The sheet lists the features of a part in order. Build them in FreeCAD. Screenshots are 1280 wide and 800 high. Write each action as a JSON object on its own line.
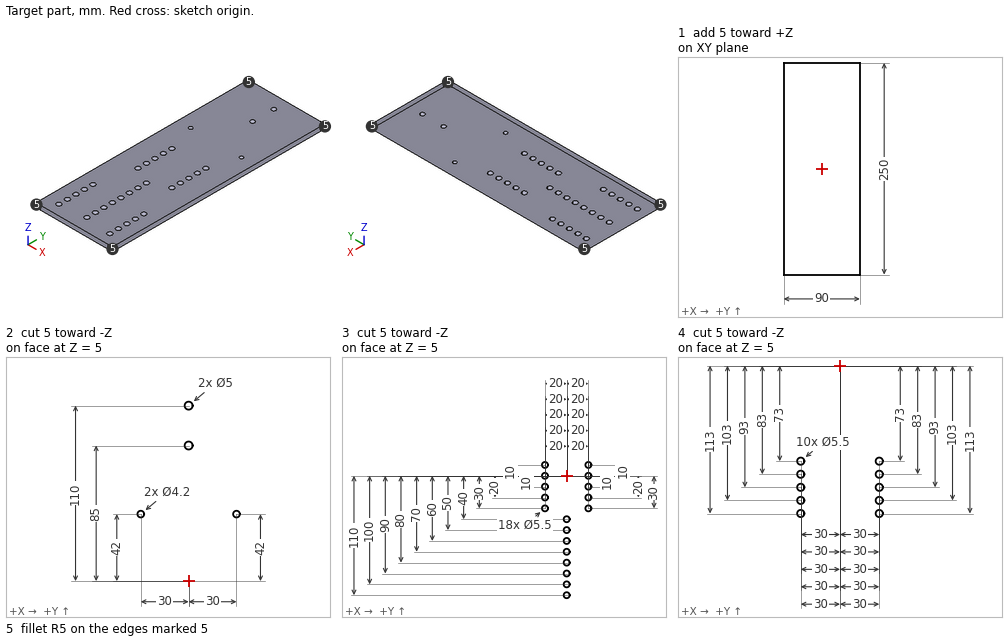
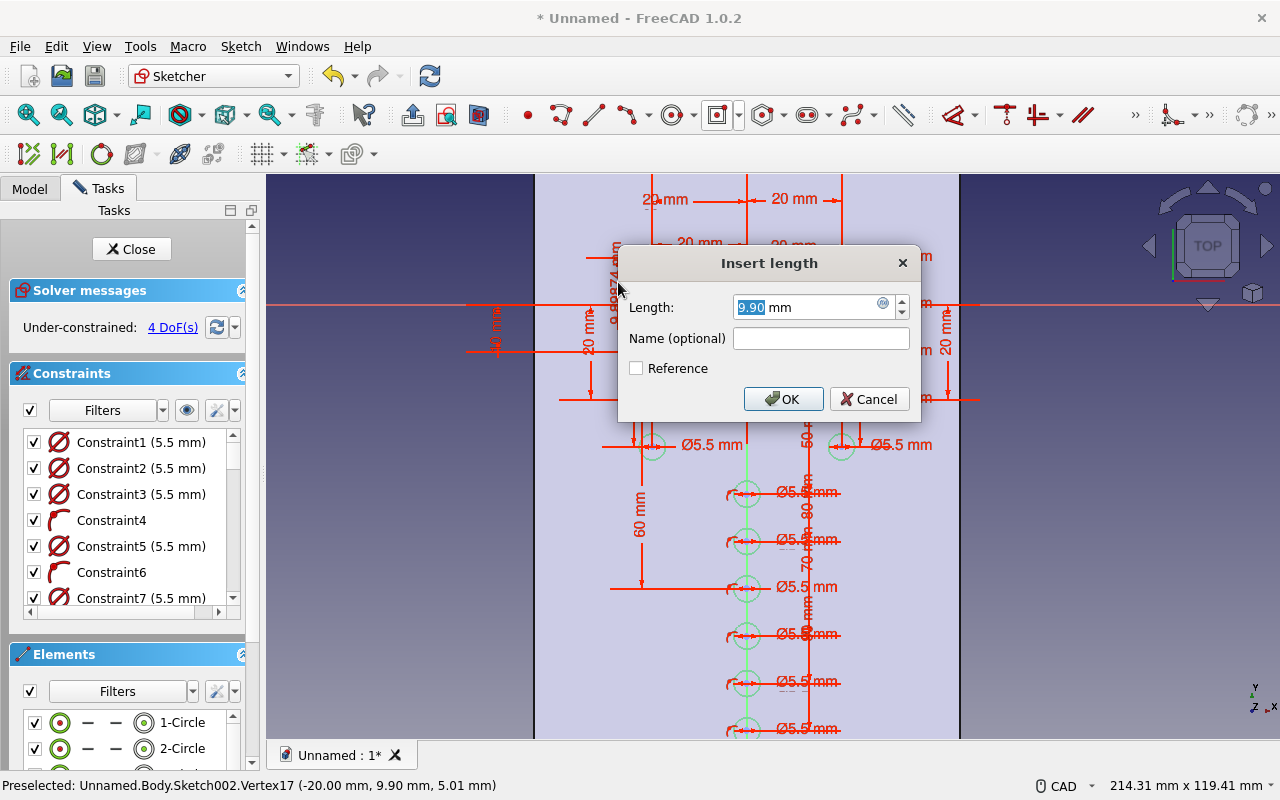
{"action": "type", "text": "10"}
{"action": "key", "text": "Return"}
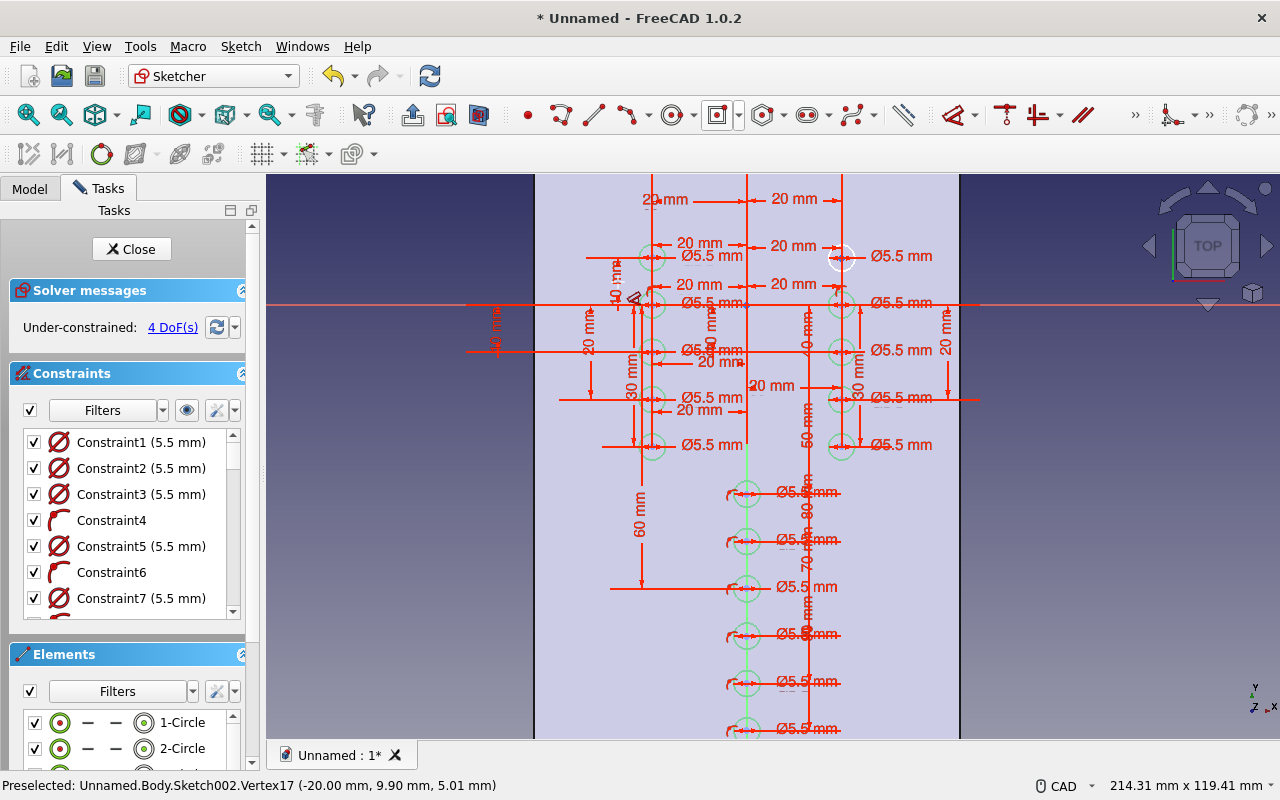
{"action": "left_click", "coordinate": [842, 258]}
{"action": "left_click", "coordinate": [794, 224]}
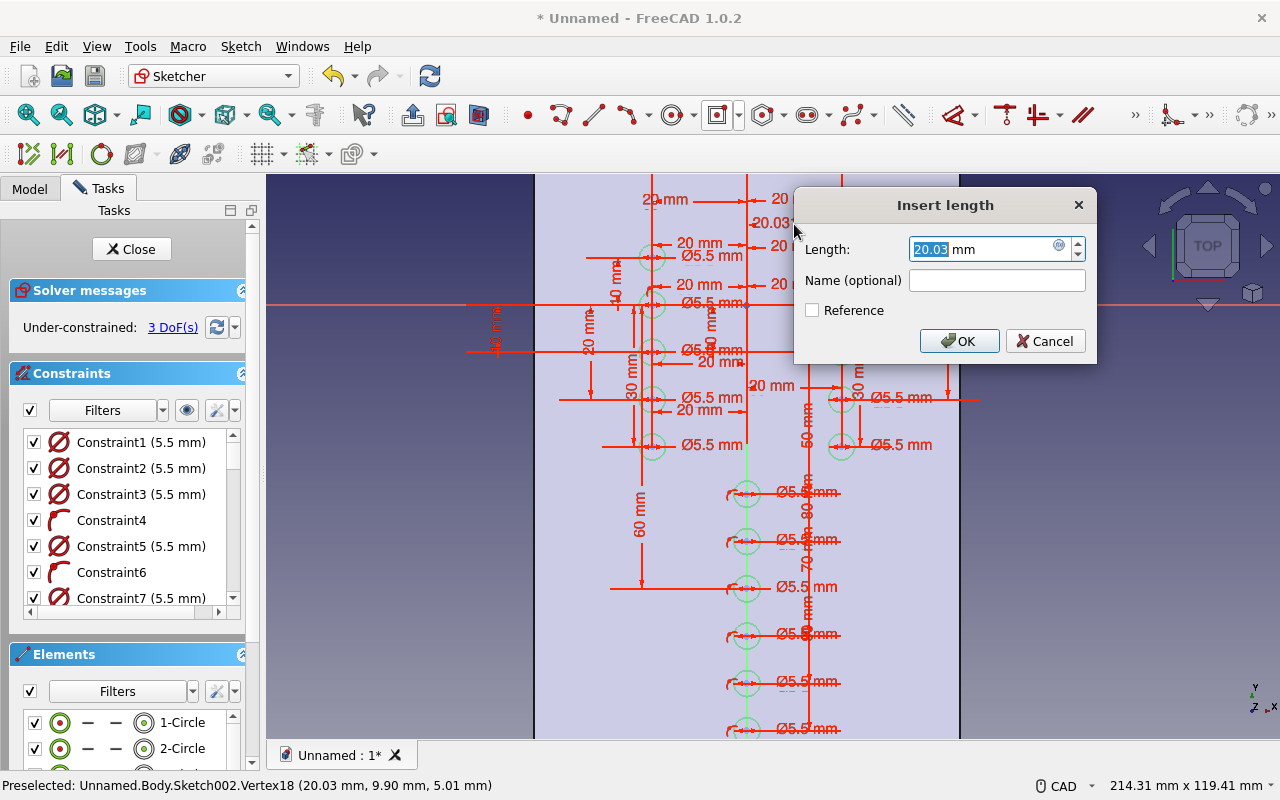
{"action": "type", "text": "20"}
{"action": "key", "text": "Return"}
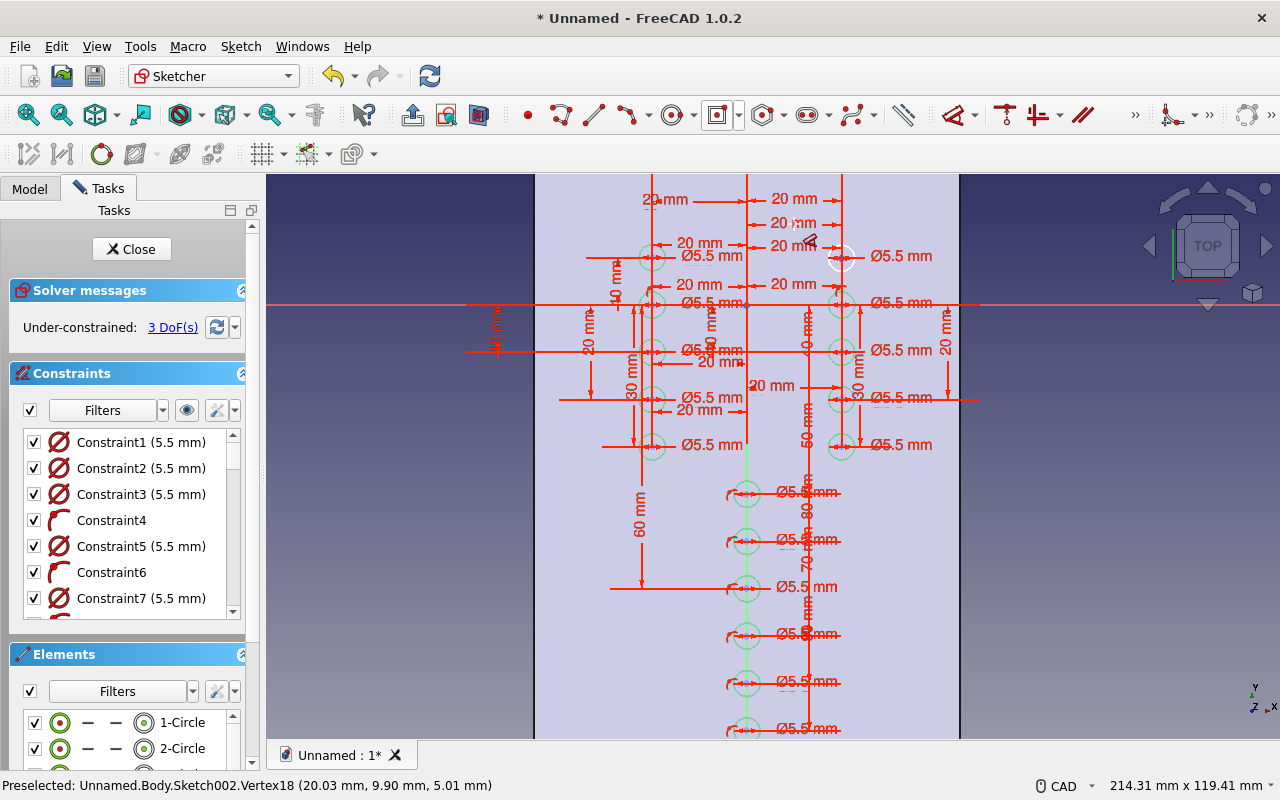
{"action": "left_click", "coordinate": [842, 258]}
{"action": "left_click", "coordinate": [876, 282]}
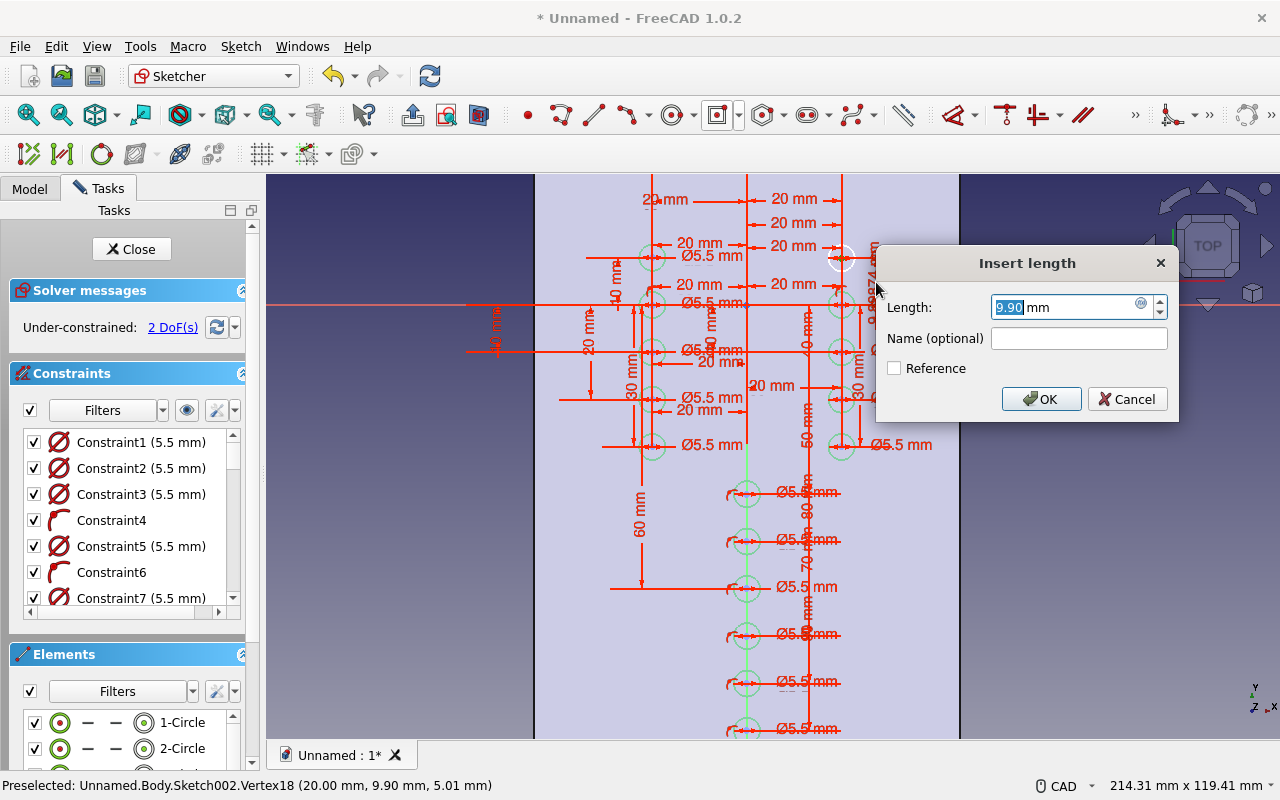
{"action": "type", "text": "10"}
{"action": "key", "text": "Return"}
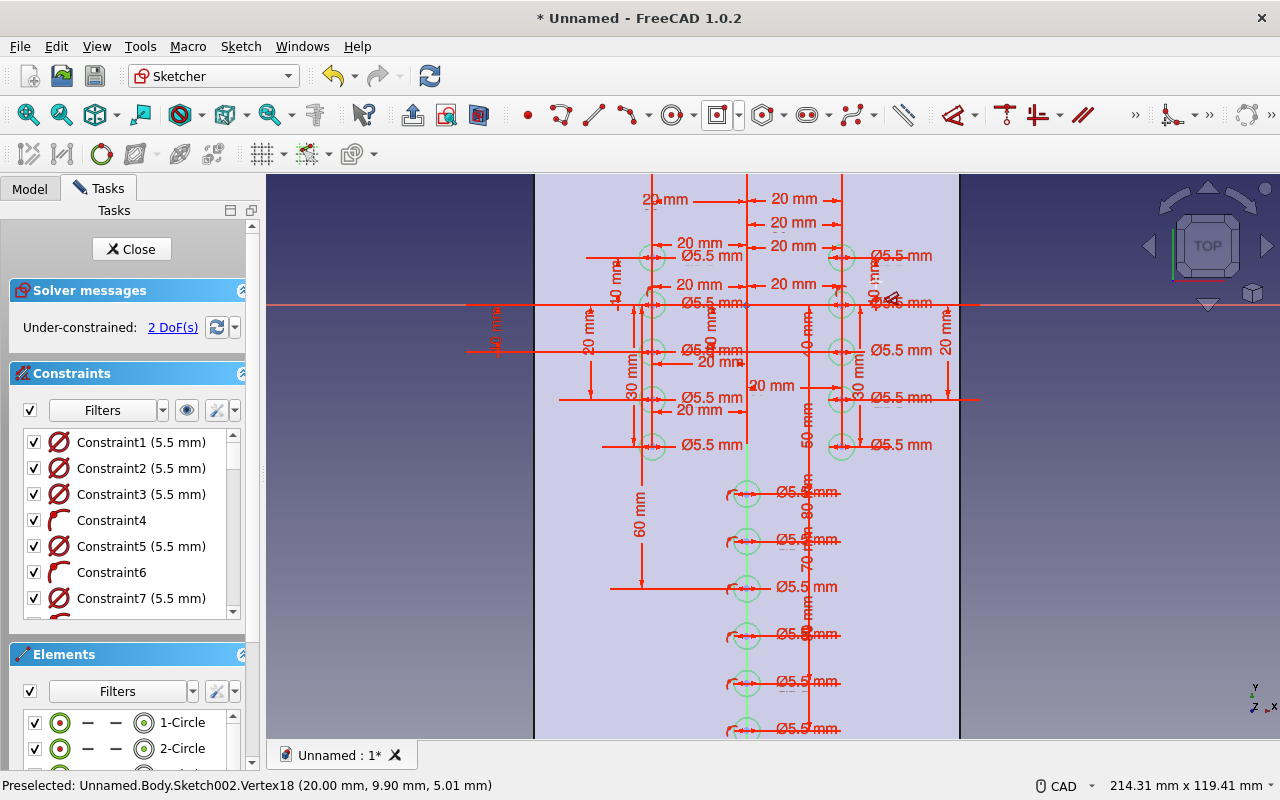
{"action": "scroll", "coordinate": [653, 353], "scroll_direction": "down", "scroll_amount": 3}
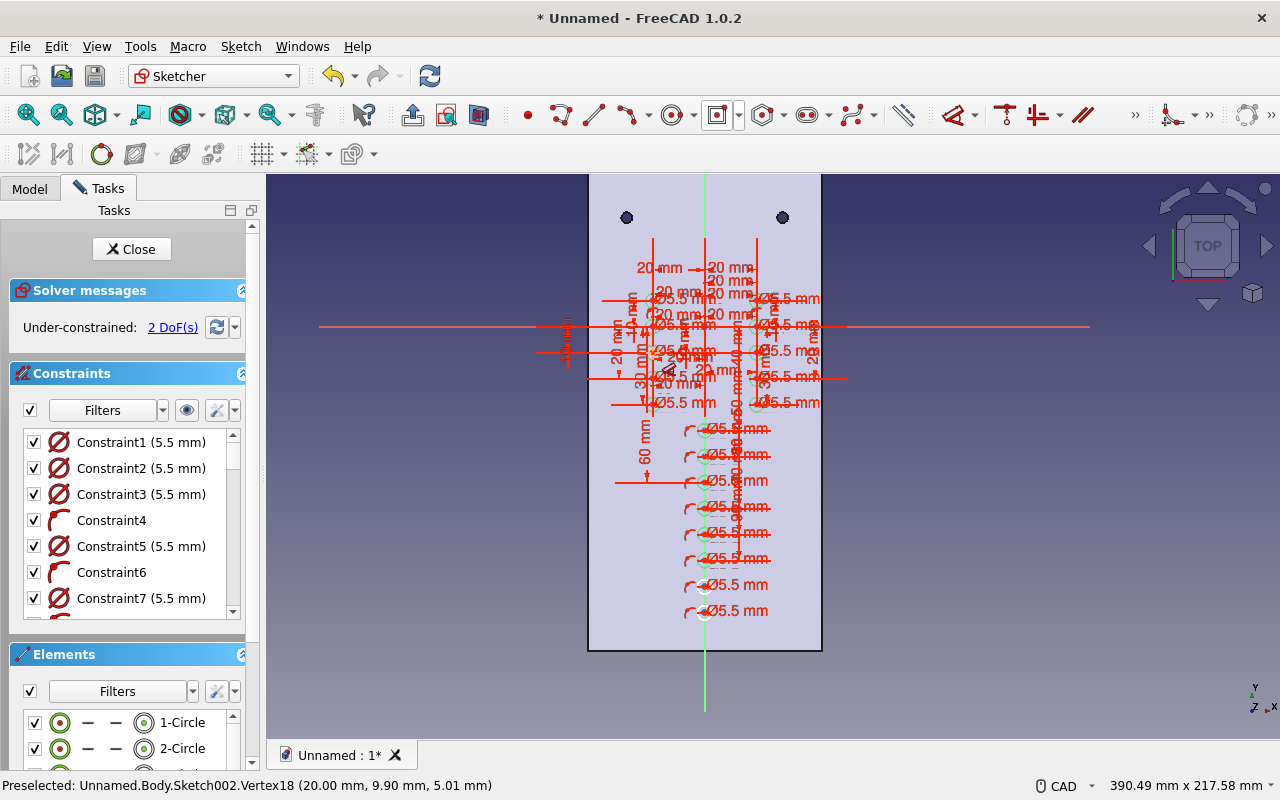
{"action": "left_click", "coordinate": [705, 587]}
{"action": "left_click", "coordinate": [739, 548]}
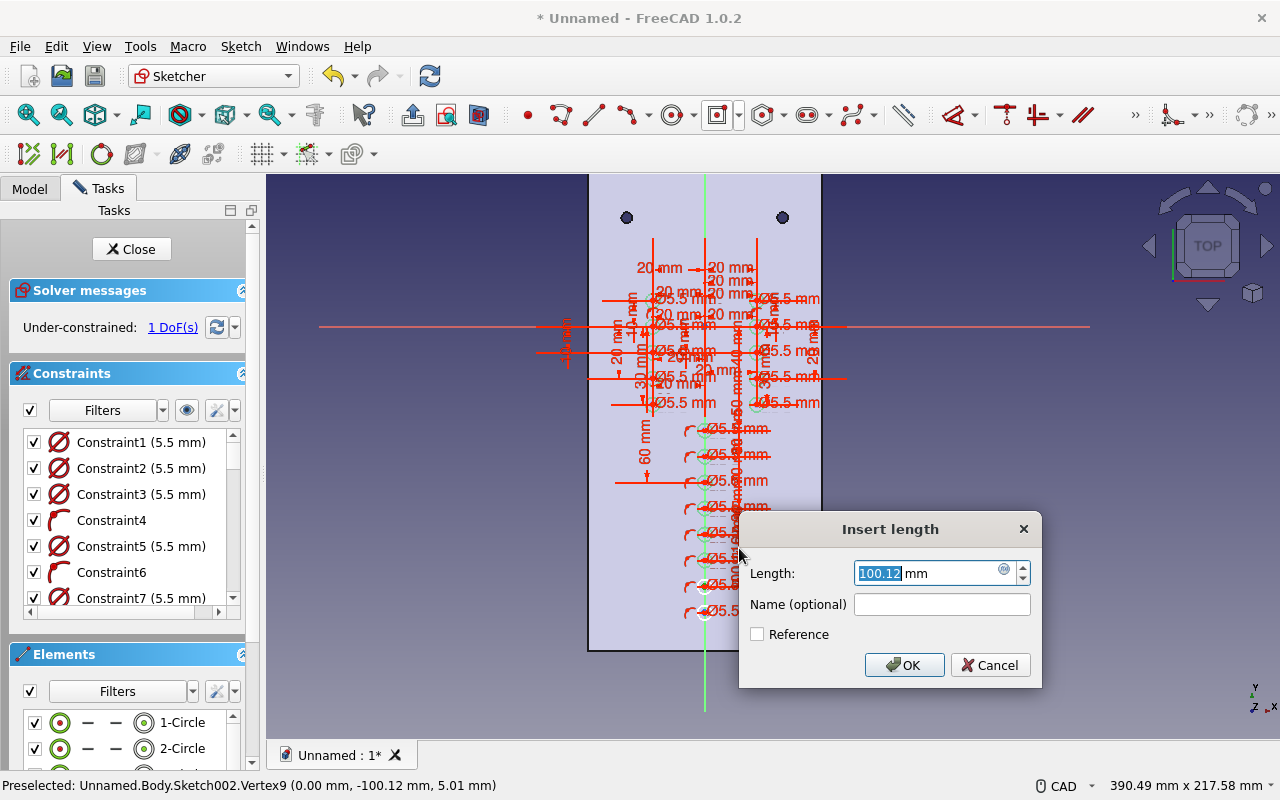
{"action": "type", "text": "100"}
{"action": "key", "text": "Return"}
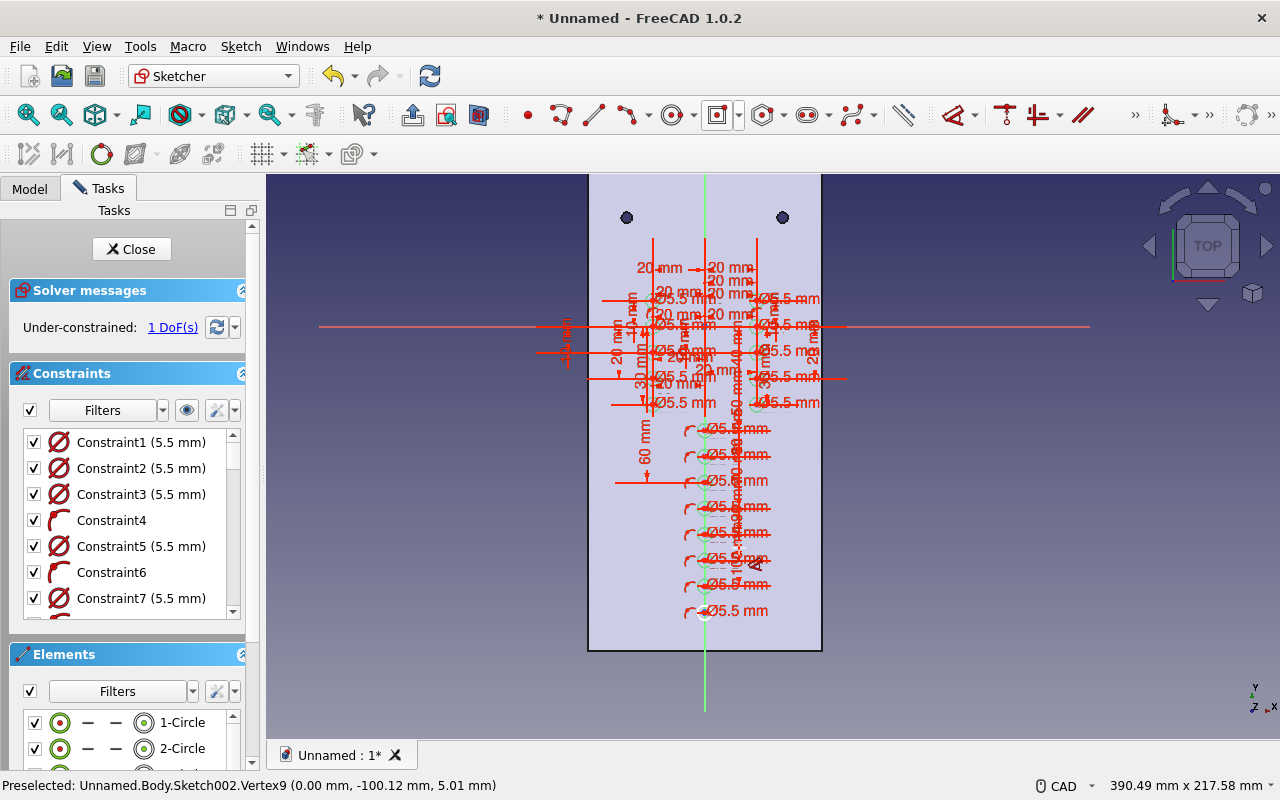
{"action": "left_click", "coordinate": [705, 613]}
{"action": "left_click", "coordinate": [739, 570]}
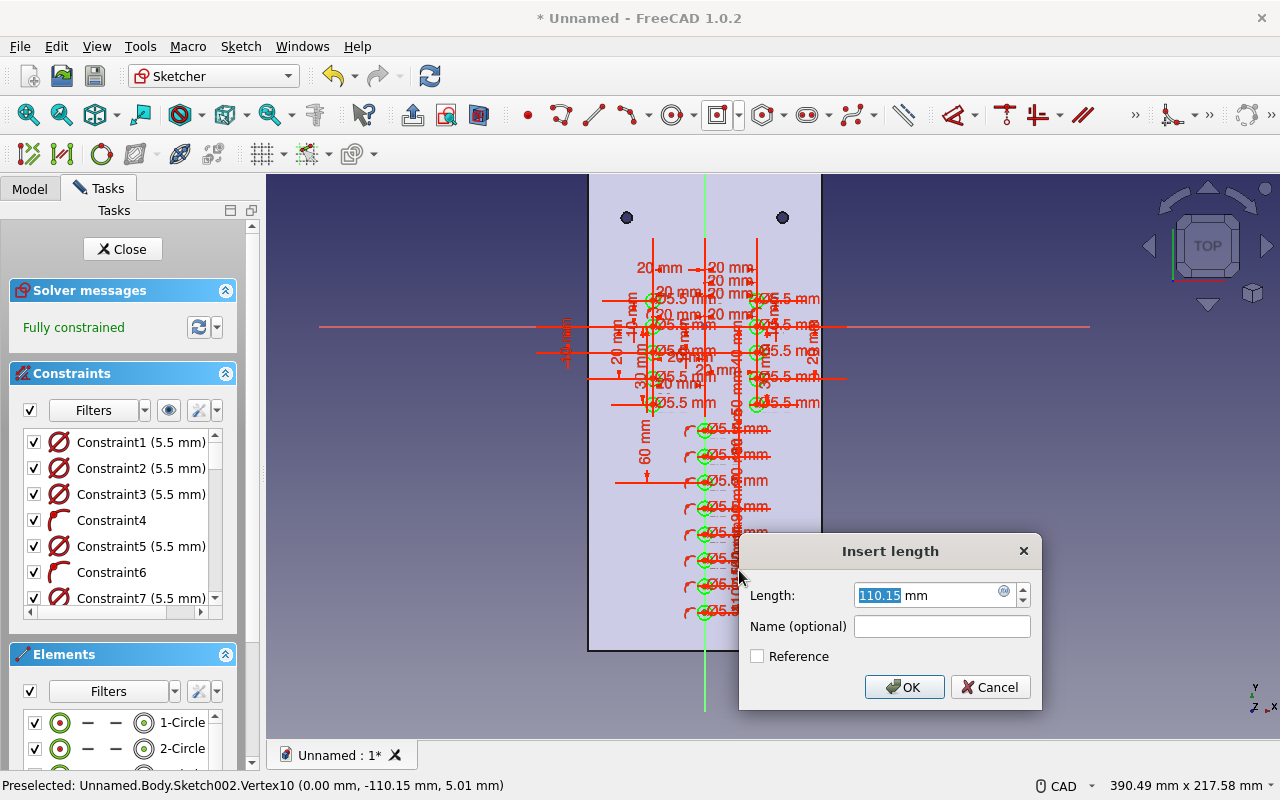
{"action": "type", "text": "110"}
{"action": "key", "text": "Return"}
{"action": "key", "text": "Escape"}